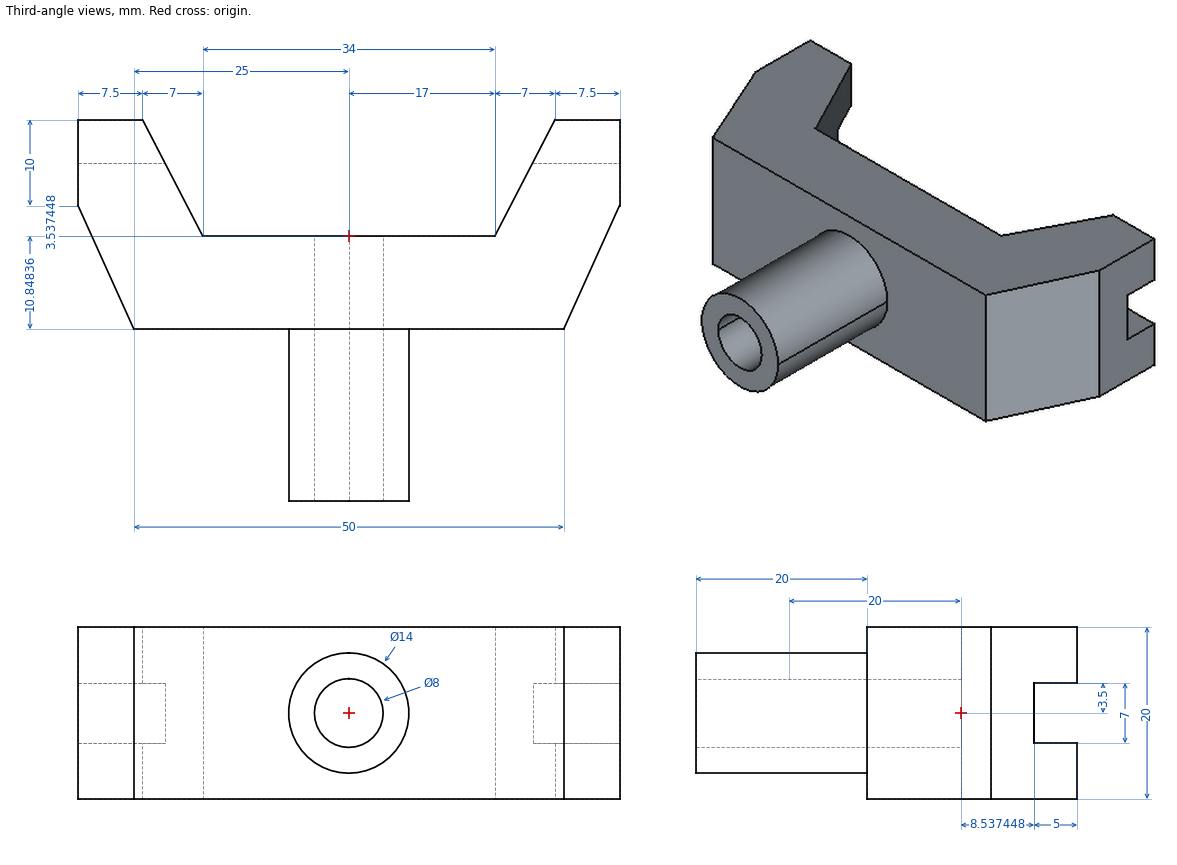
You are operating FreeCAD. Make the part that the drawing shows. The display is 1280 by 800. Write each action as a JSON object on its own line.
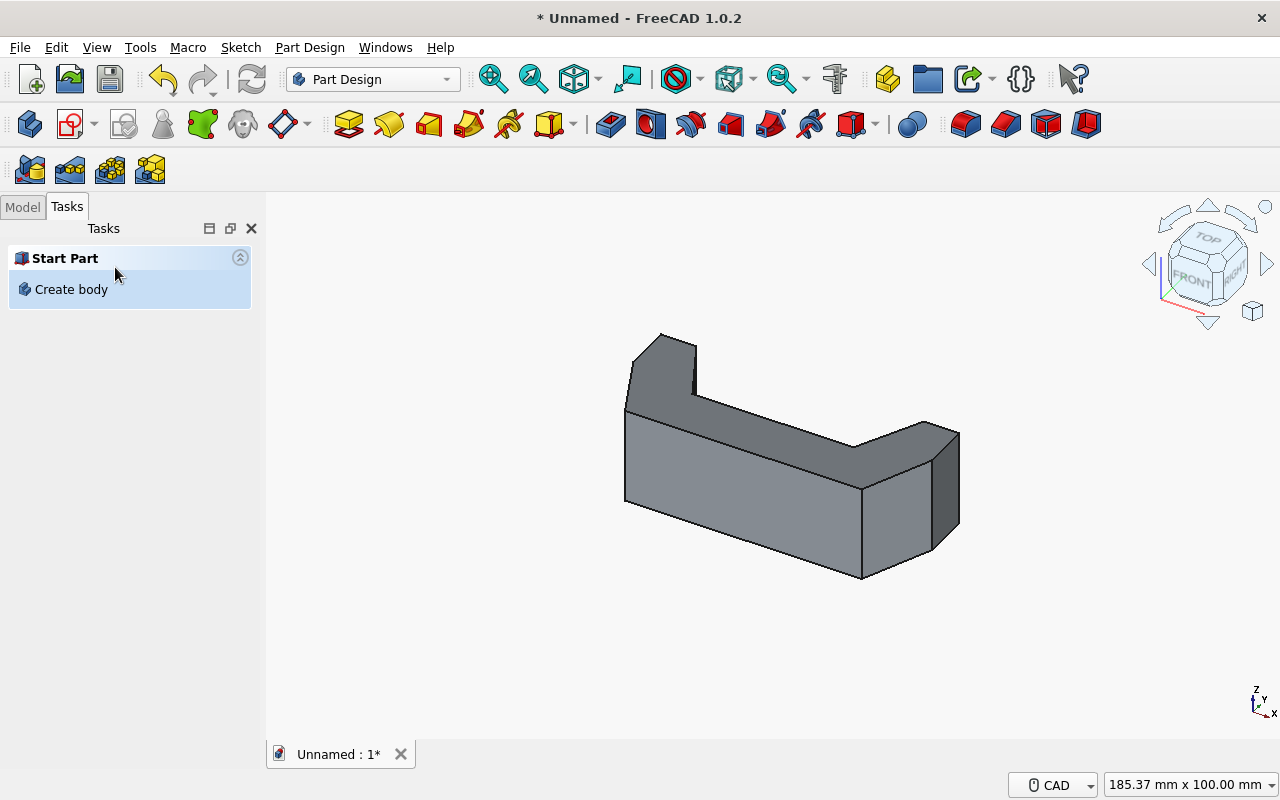
{"action": "key", "text": "6"}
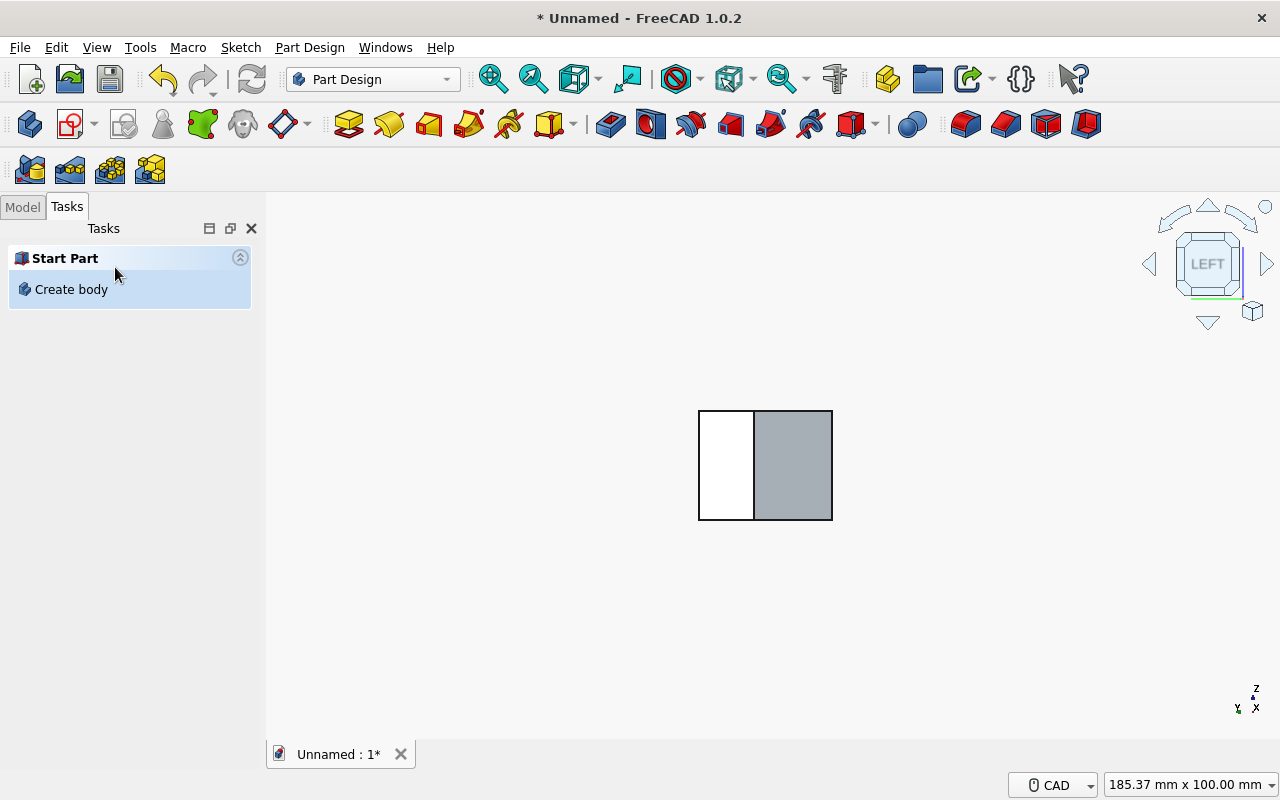
{"action": "left_click", "coordinate": [494, 80]}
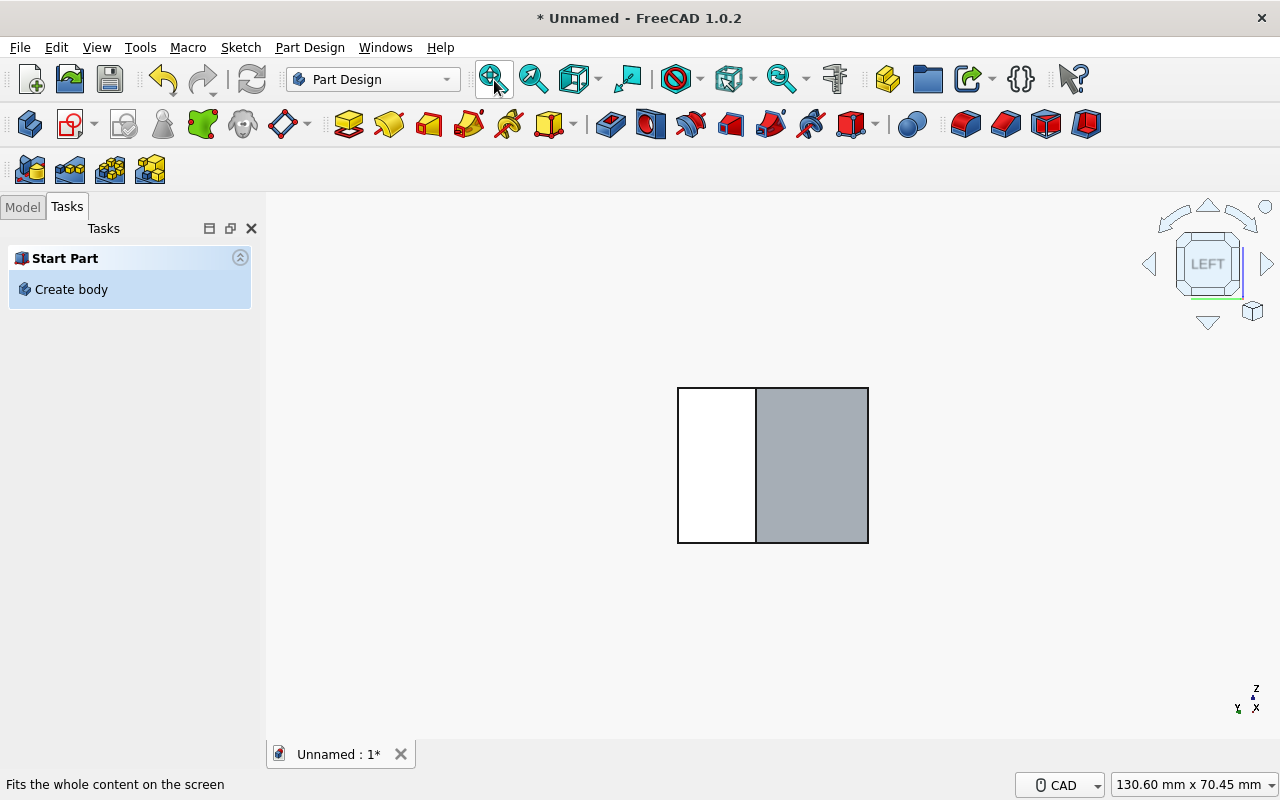
{"action": "left_click", "coordinate": [717, 442]}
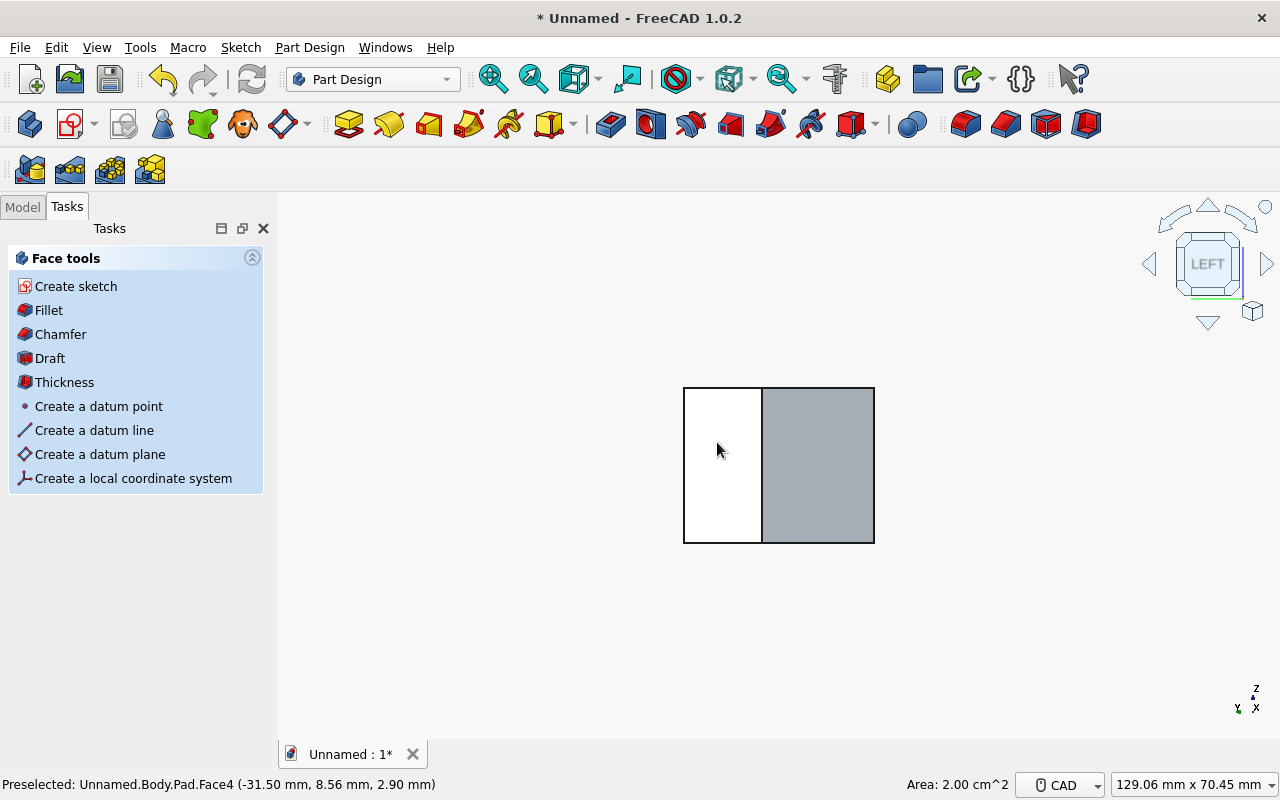
{"action": "left_click", "coordinate": [70, 124]}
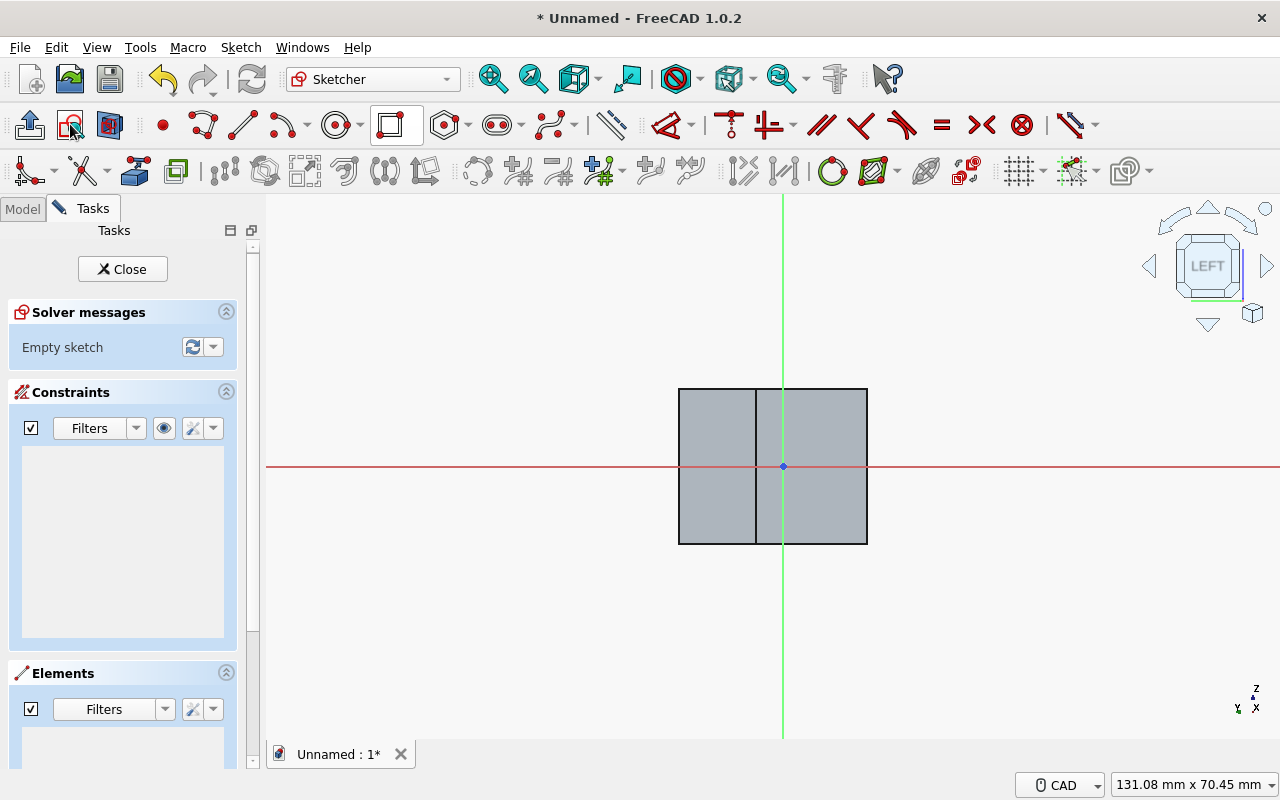
{"action": "scroll", "coordinate": [736, 467], "scroll_direction": "up", "scroll_amount": 9}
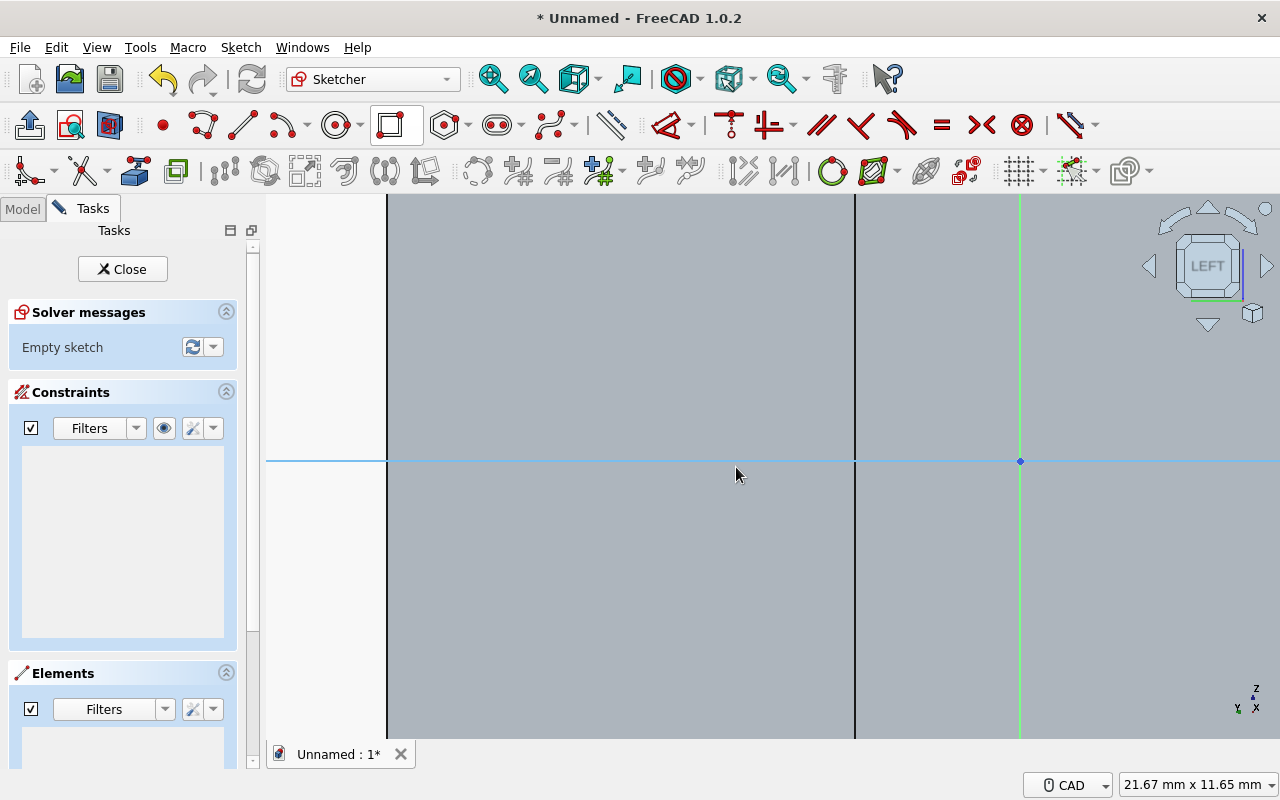
{"action": "left_click", "coordinate": [390, 126]}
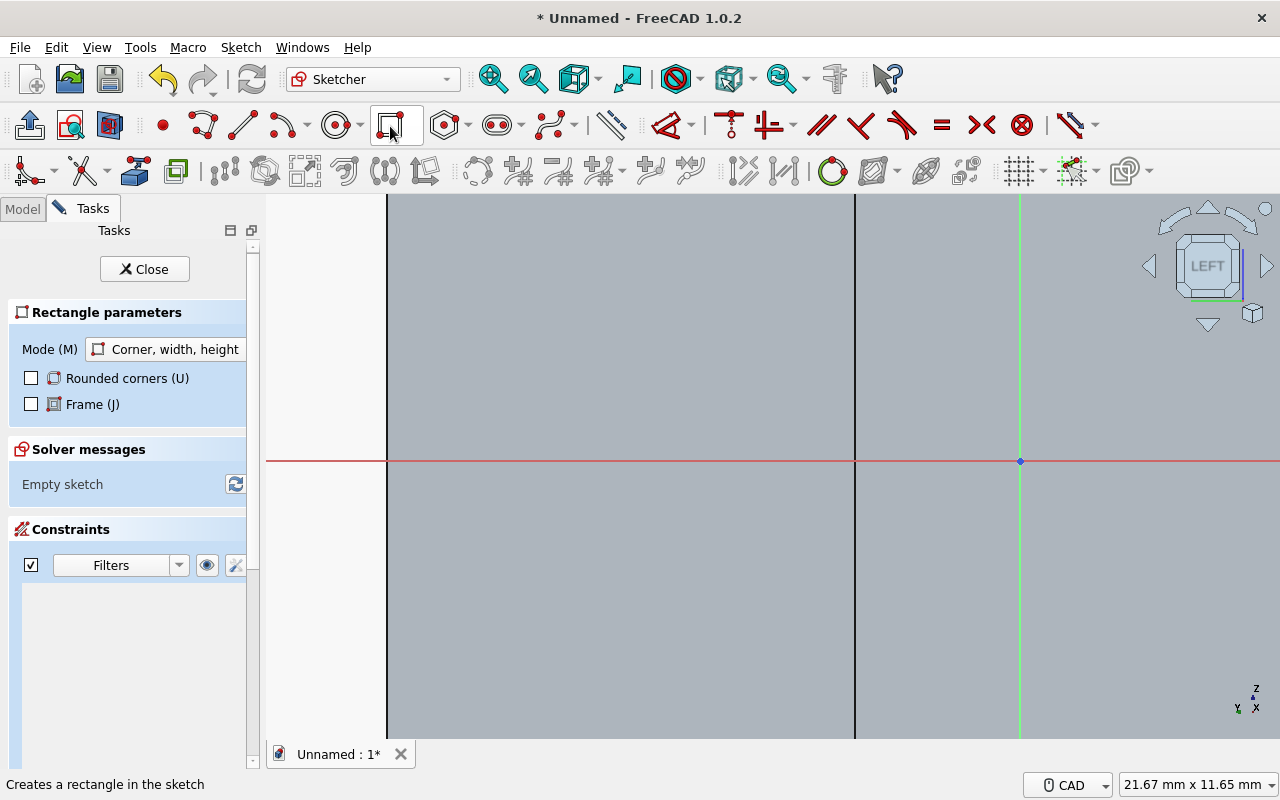
{"action": "left_click", "coordinate": [387, 298]}
{"action": "mouse_move", "coordinate": [621, 625]}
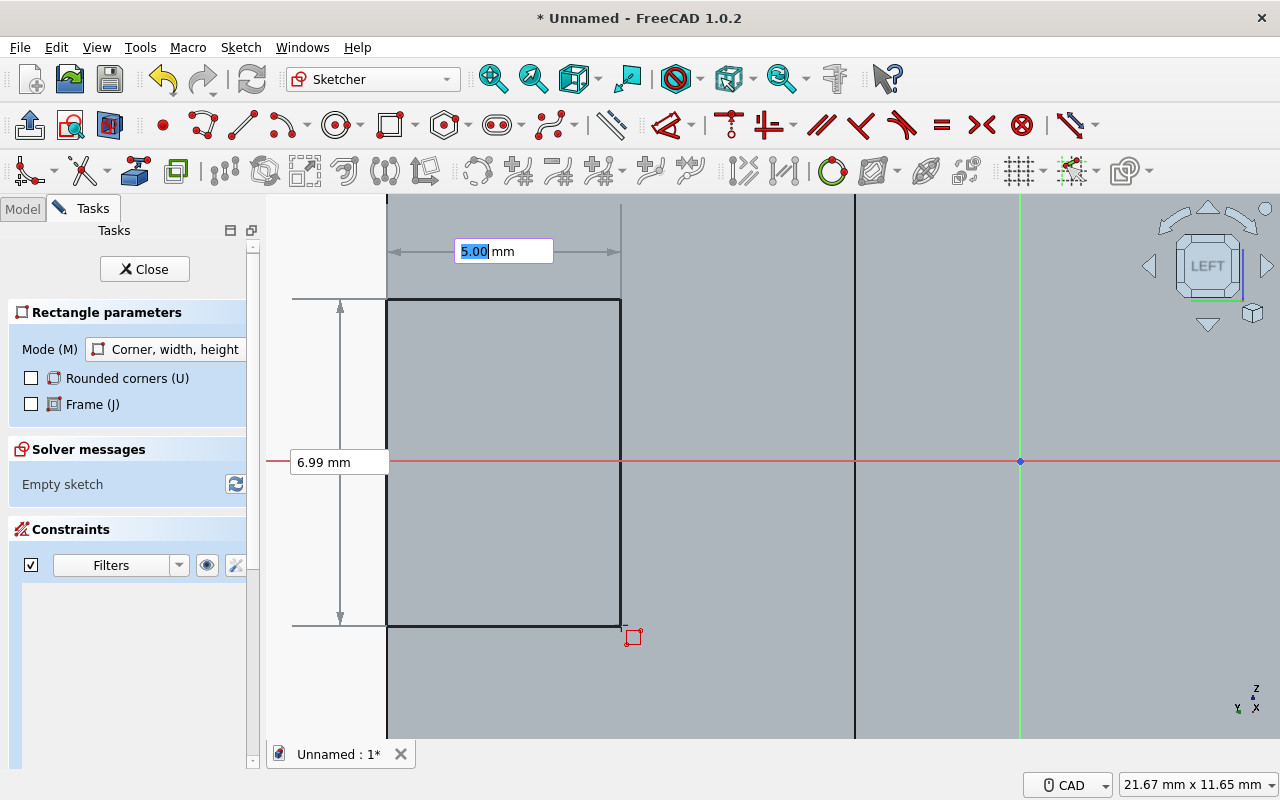
{"action": "type", "text": "5"}
{"action": "key", "text": "Tab"}
{"action": "type", "text": "7"}
{"action": "key", "text": "Return"}
{"action": "key", "text": "Escape"}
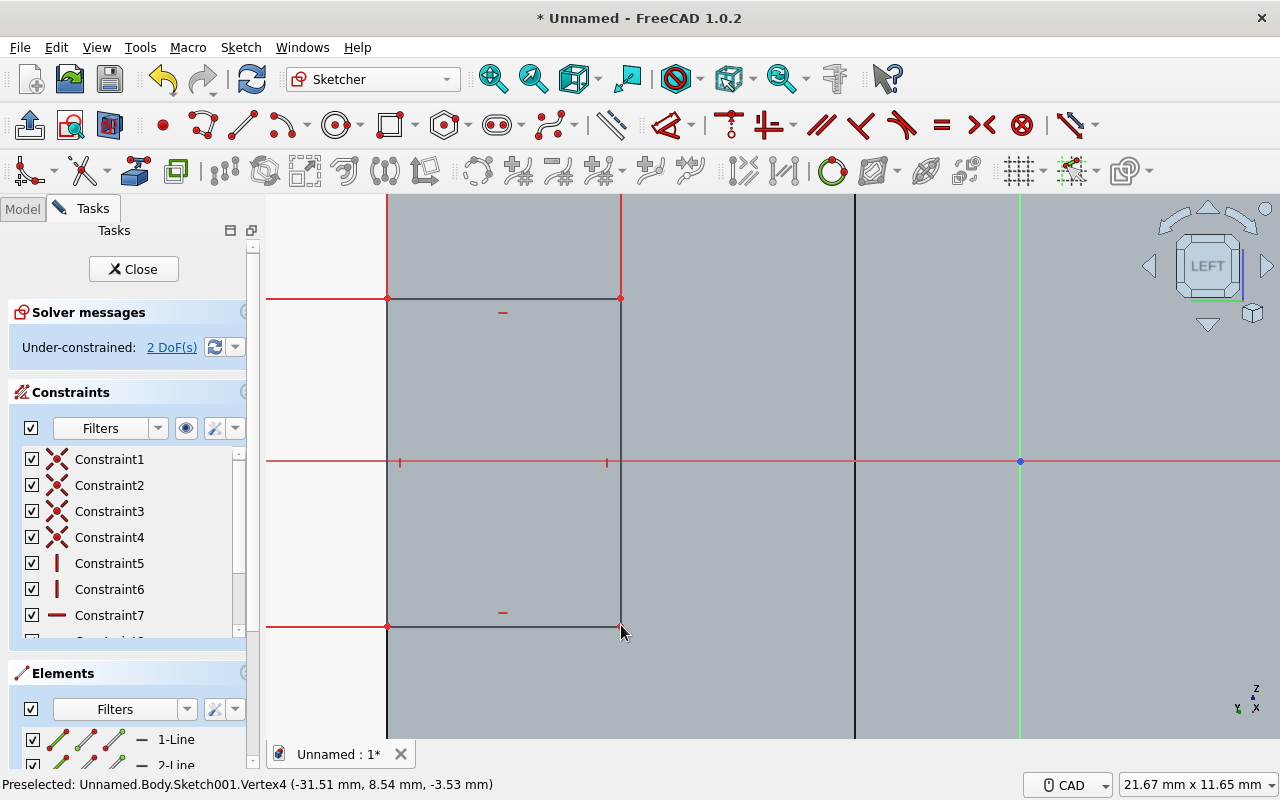
{"action": "left_click", "coordinate": [666, 126]}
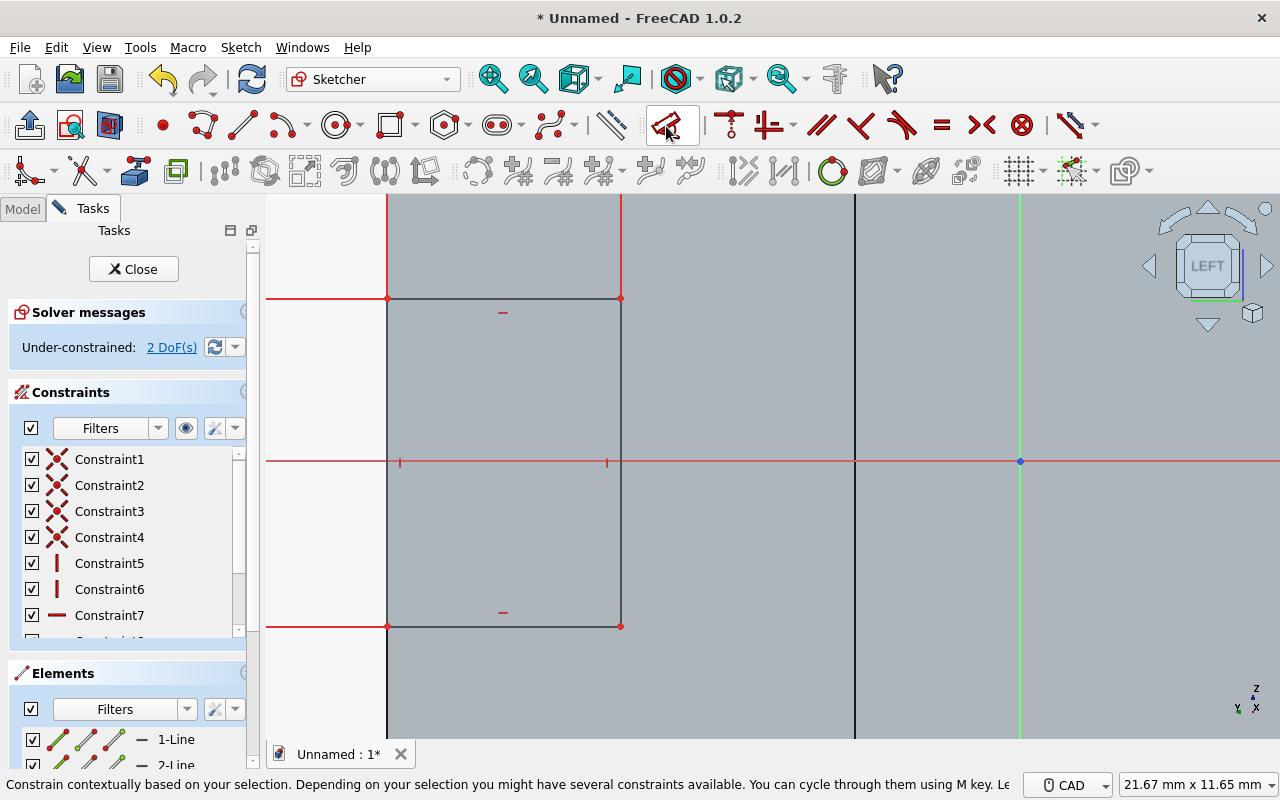
{"action": "left_click", "coordinate": [387, 299]}
{"action": "left_click", "coordinate": [1054, 380]}